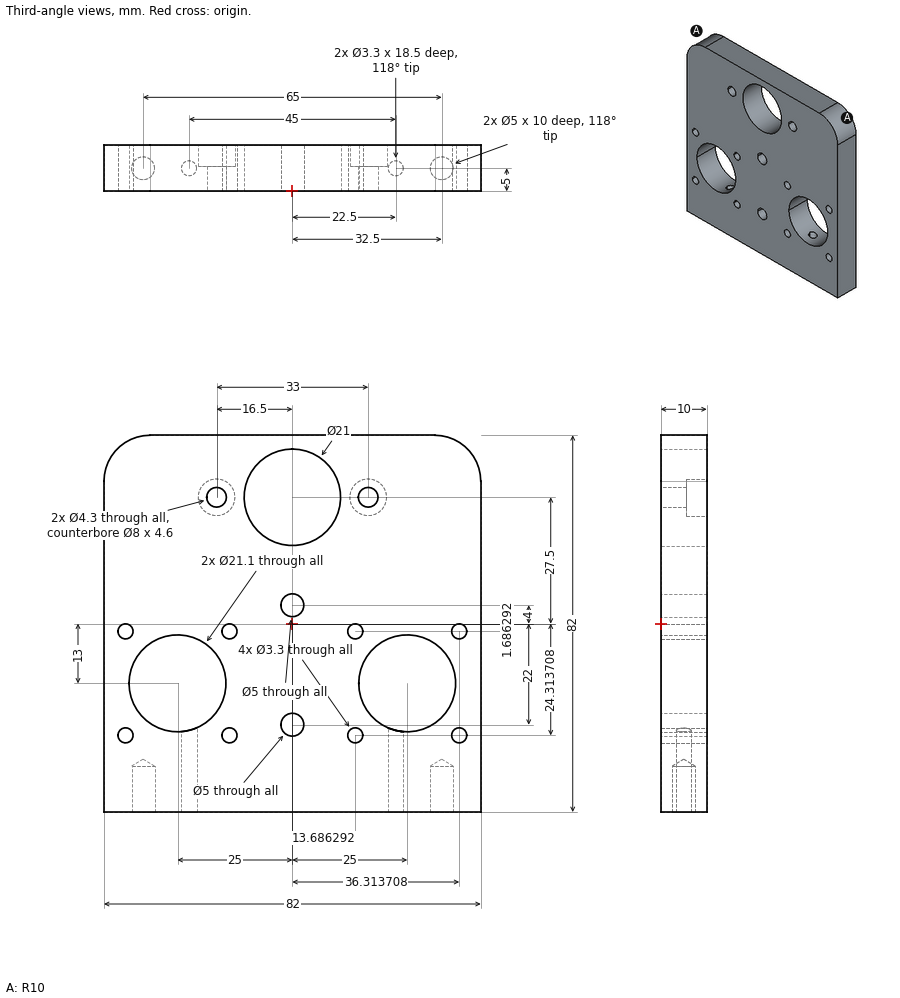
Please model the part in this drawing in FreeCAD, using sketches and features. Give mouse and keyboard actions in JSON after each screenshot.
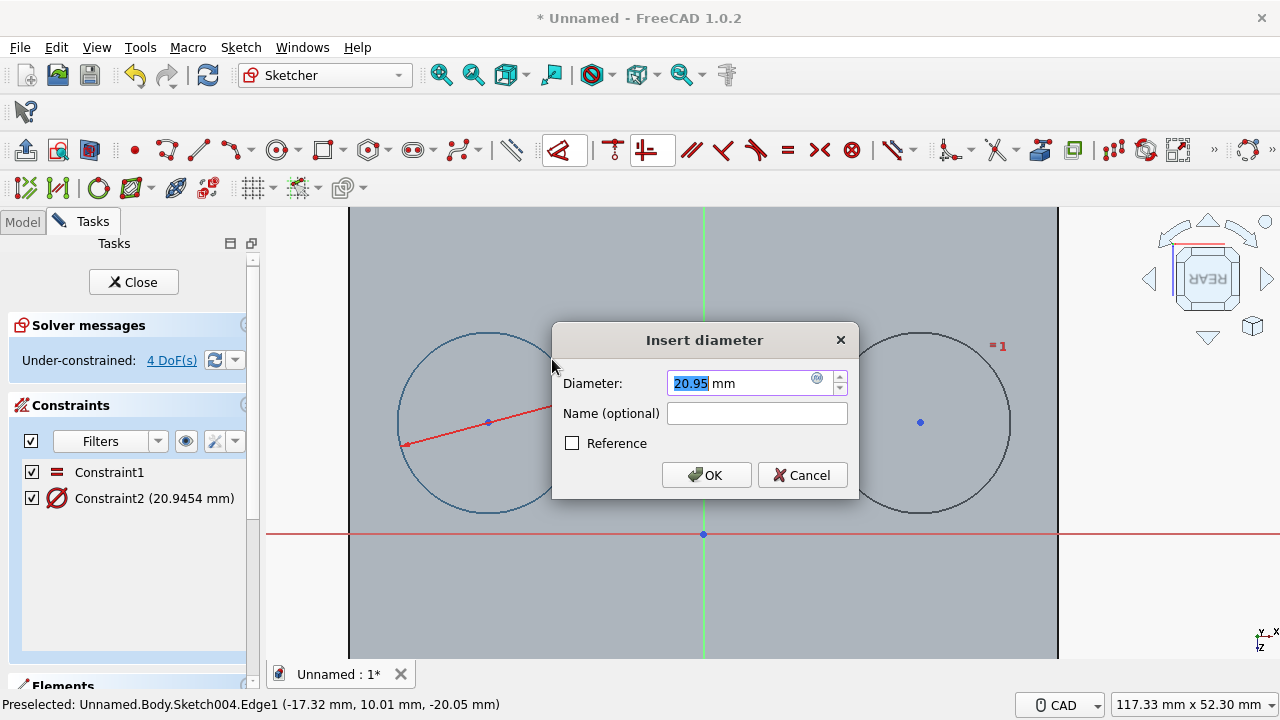
{"action": "type", "text": "21.1"}
{"action": "key", "text": "Return"}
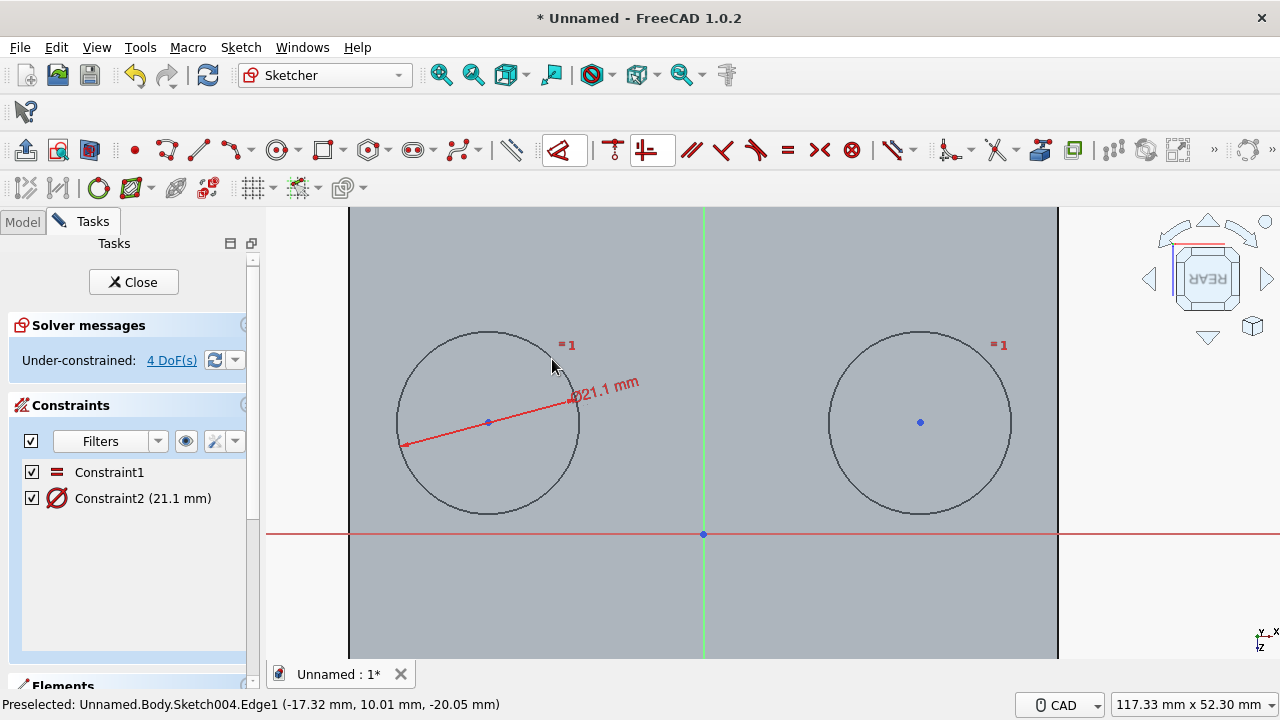
{"action": "left_click", "coordinate": [488, 423]}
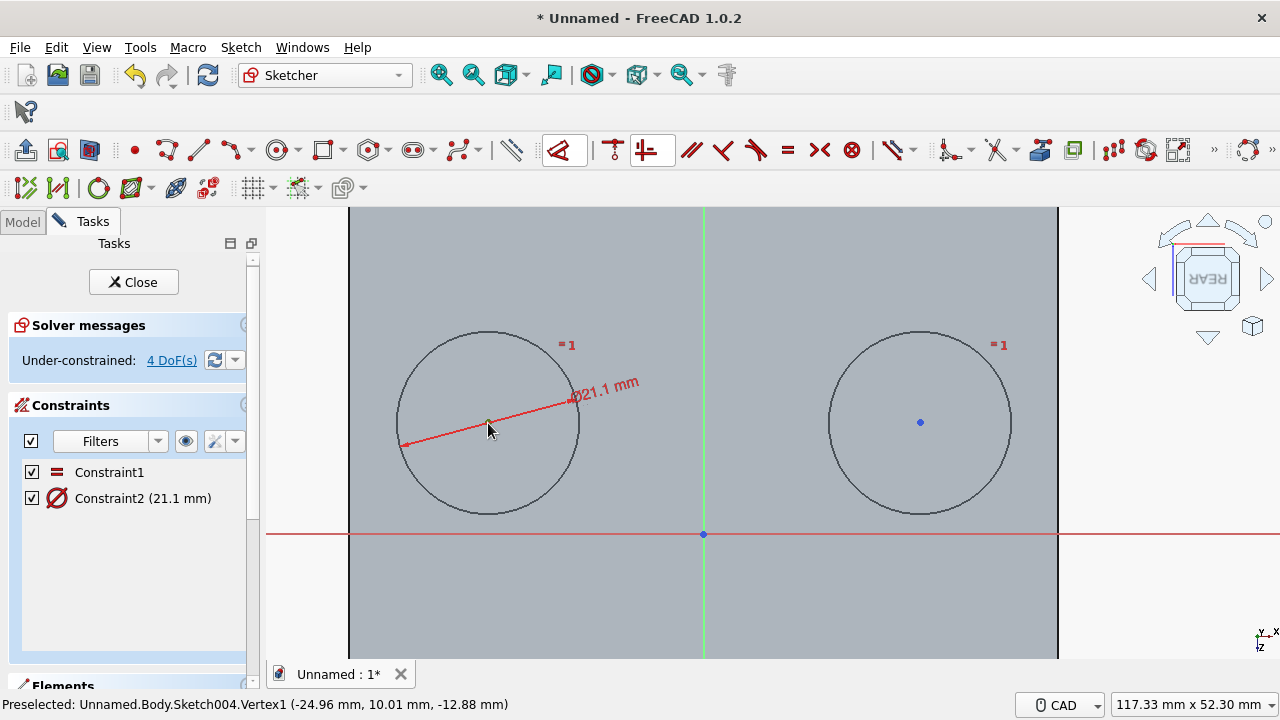
{"action": "key", "text": "l"}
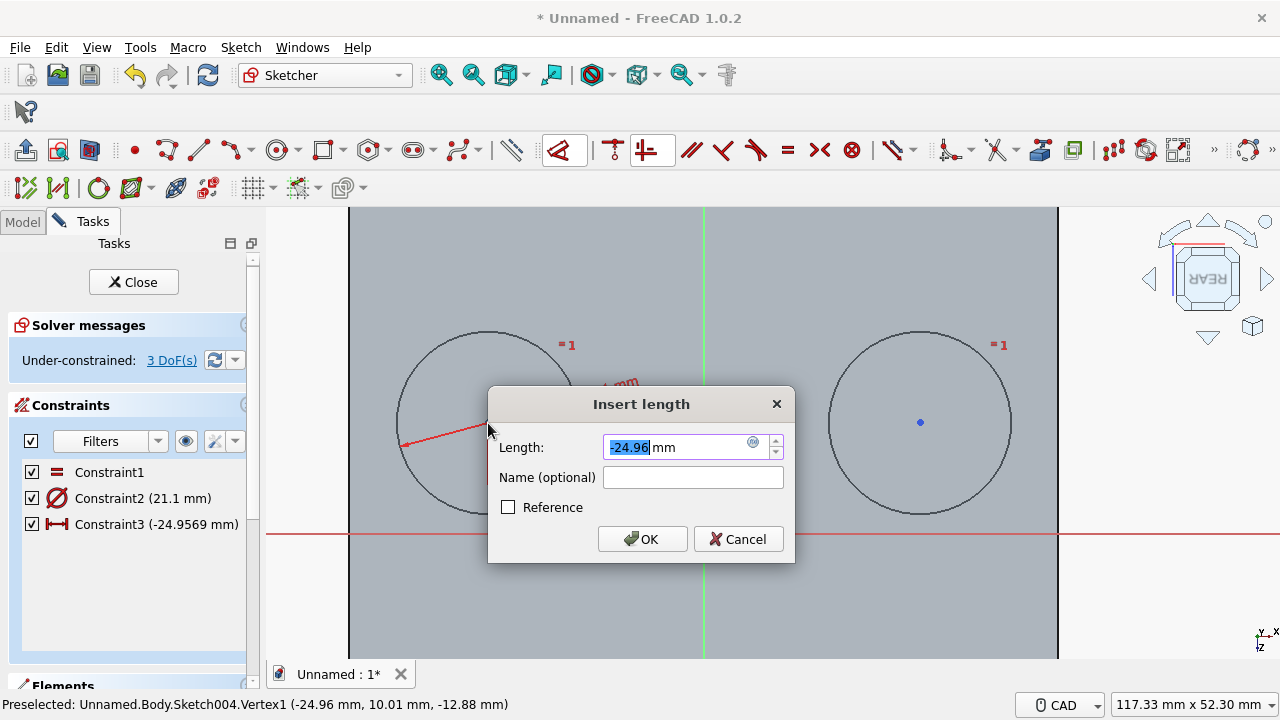
{"action": "type", "text": "-25"}
{"action": "key", "text": "Return"}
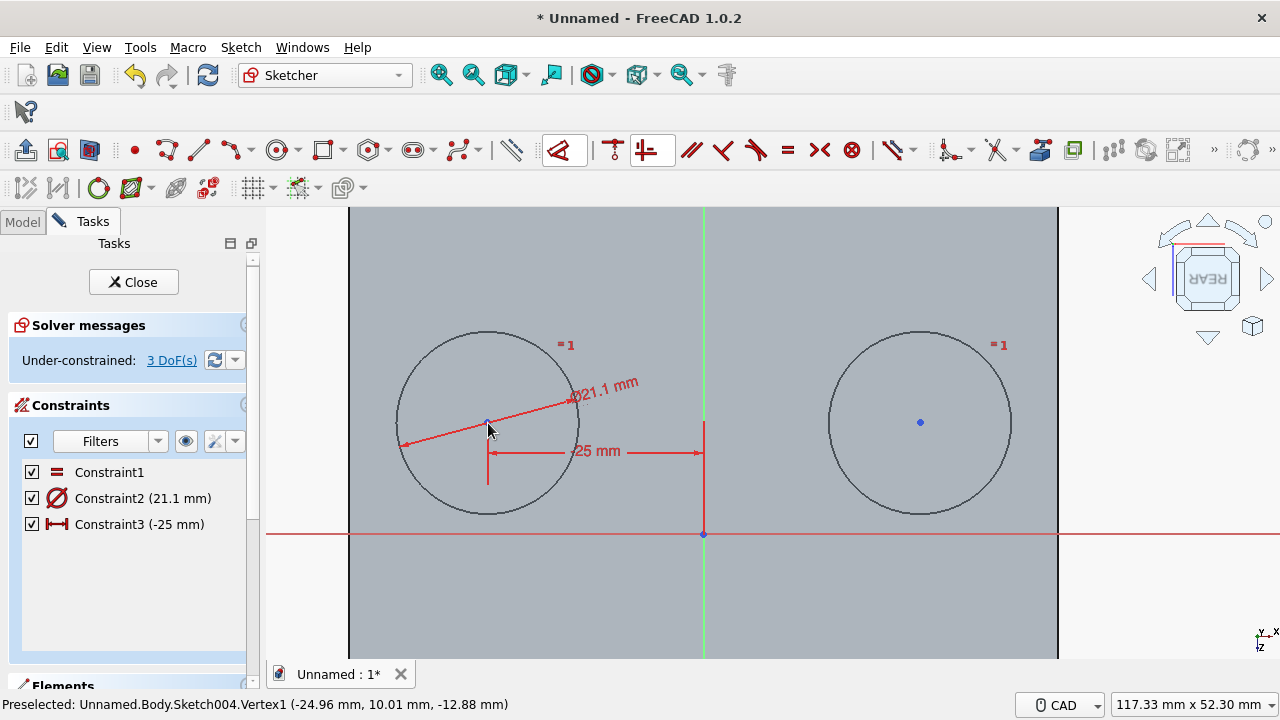
{"action": "left_click", "coordinate": [488, 423]}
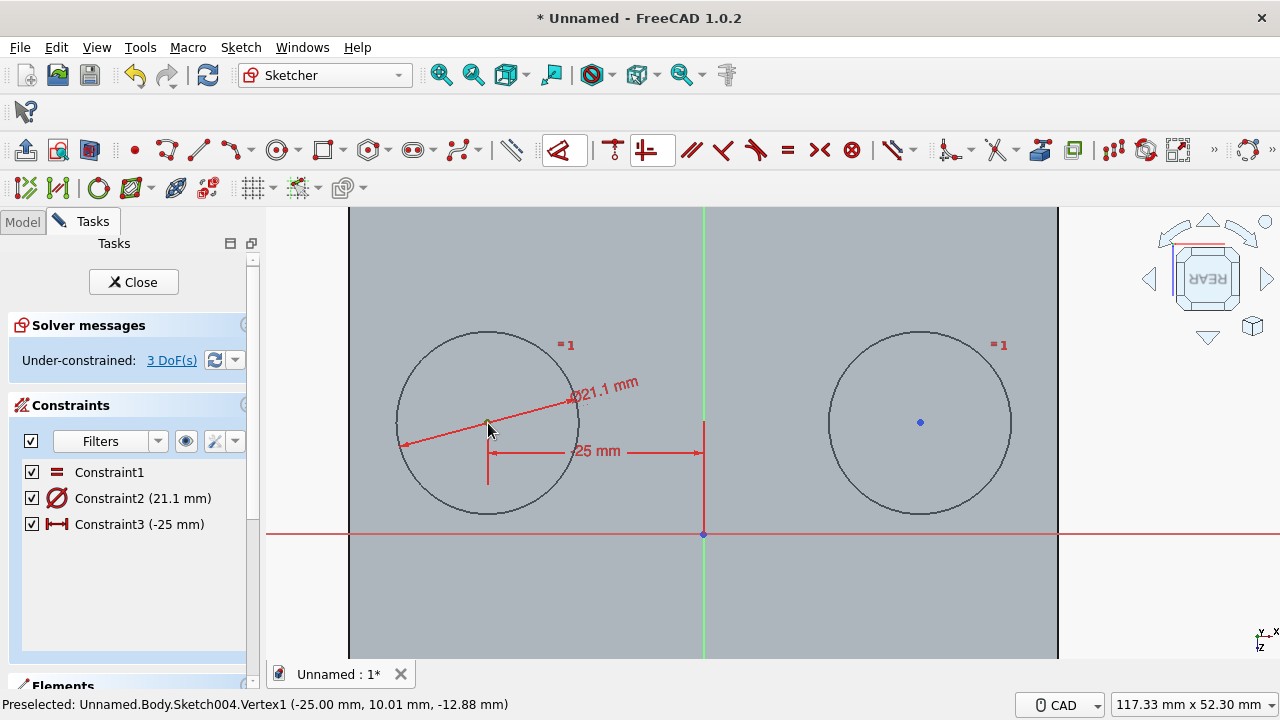
{"action": "key", "text": "i"}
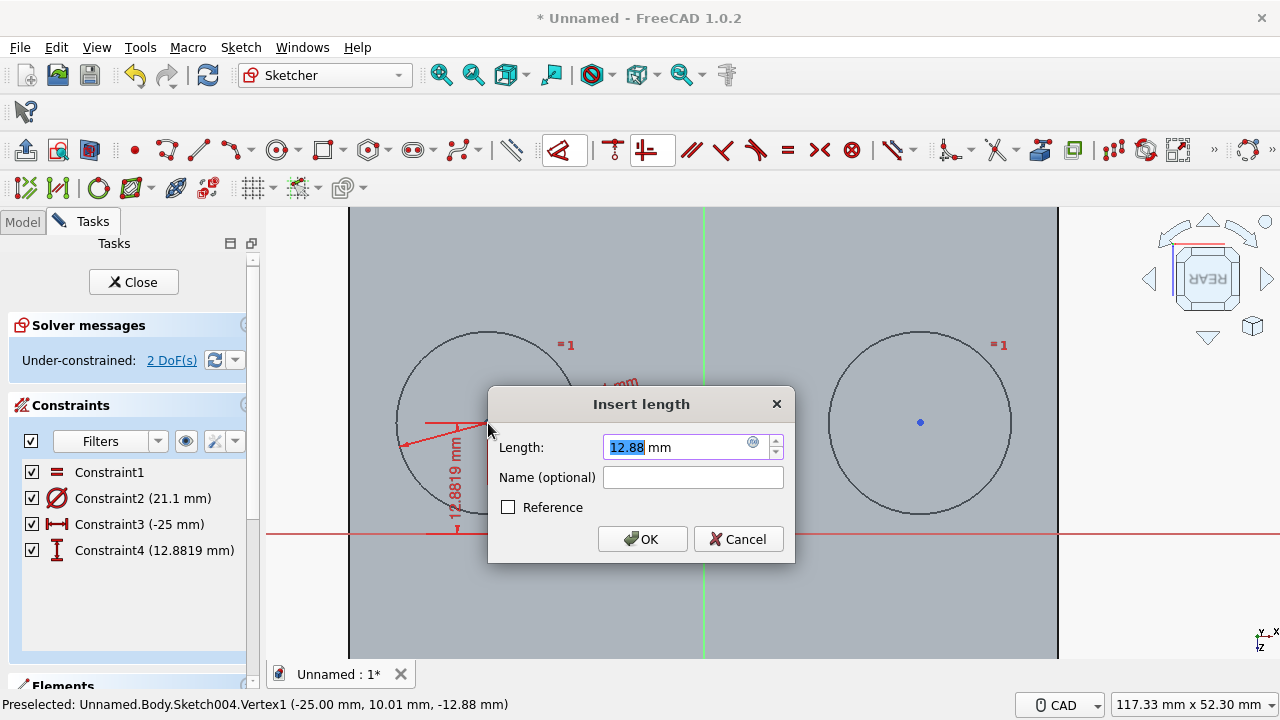
{"action": "type", "text": "13"}
{"action": "key", "text": "Return"}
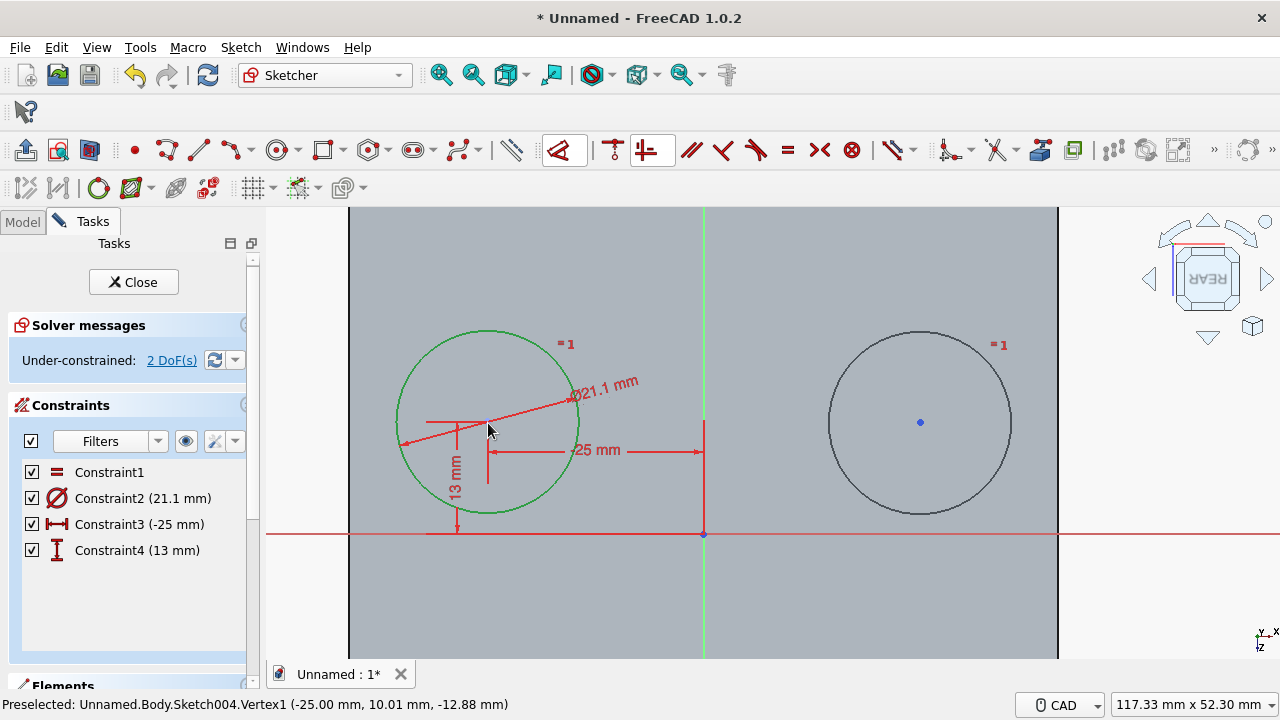
{"action": "left_click", "coordinate": [920, 423]}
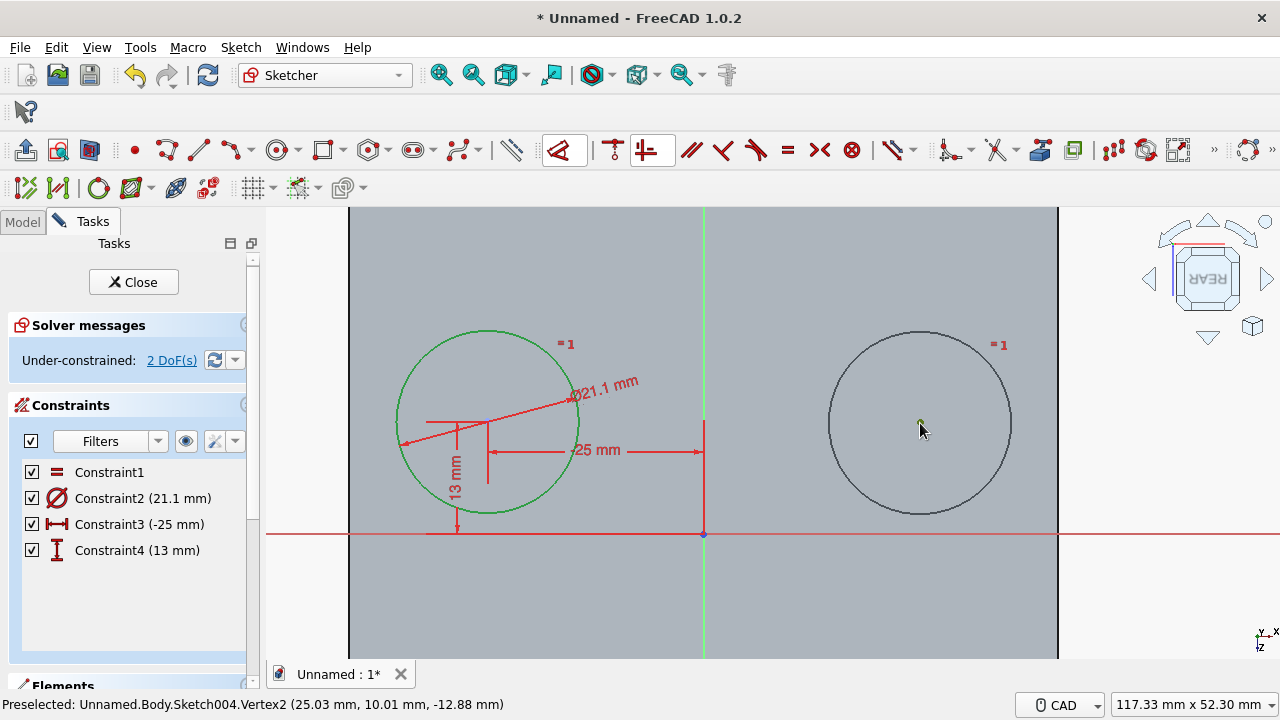
{"action": "key", "text": "l"}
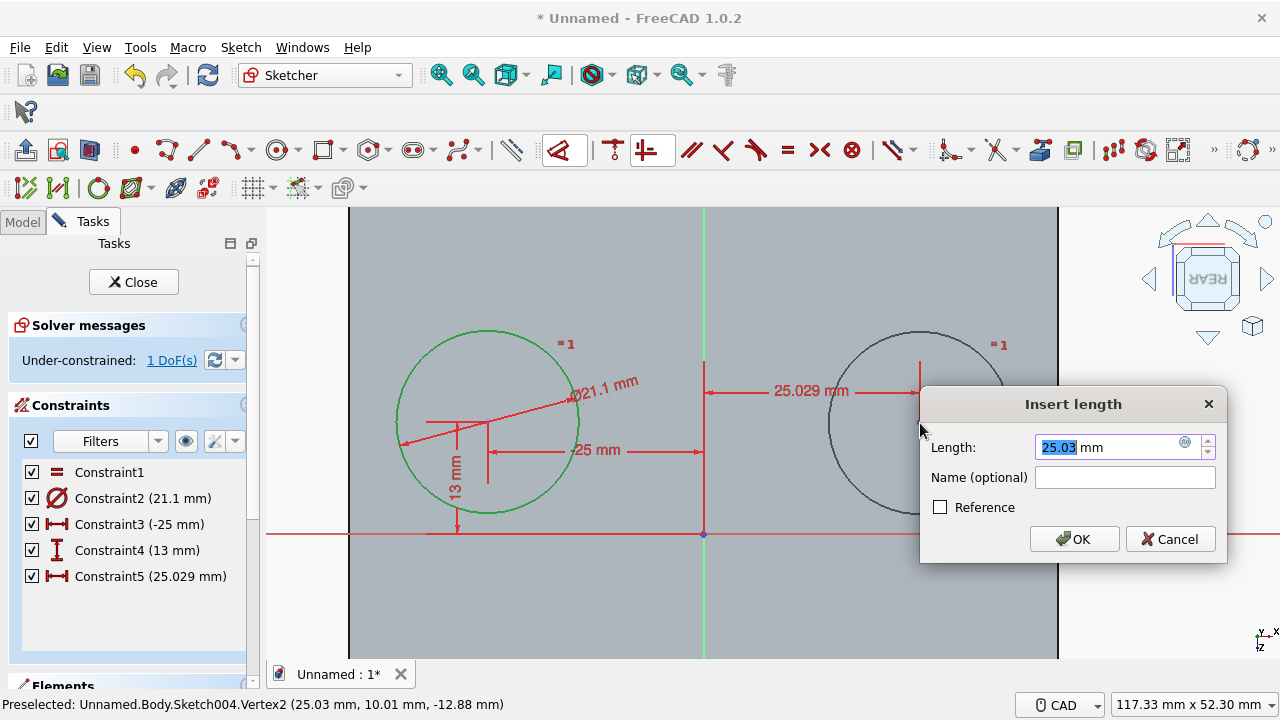
{"action": "type", "text": "25"}
{"action": "key", "text": "Return"}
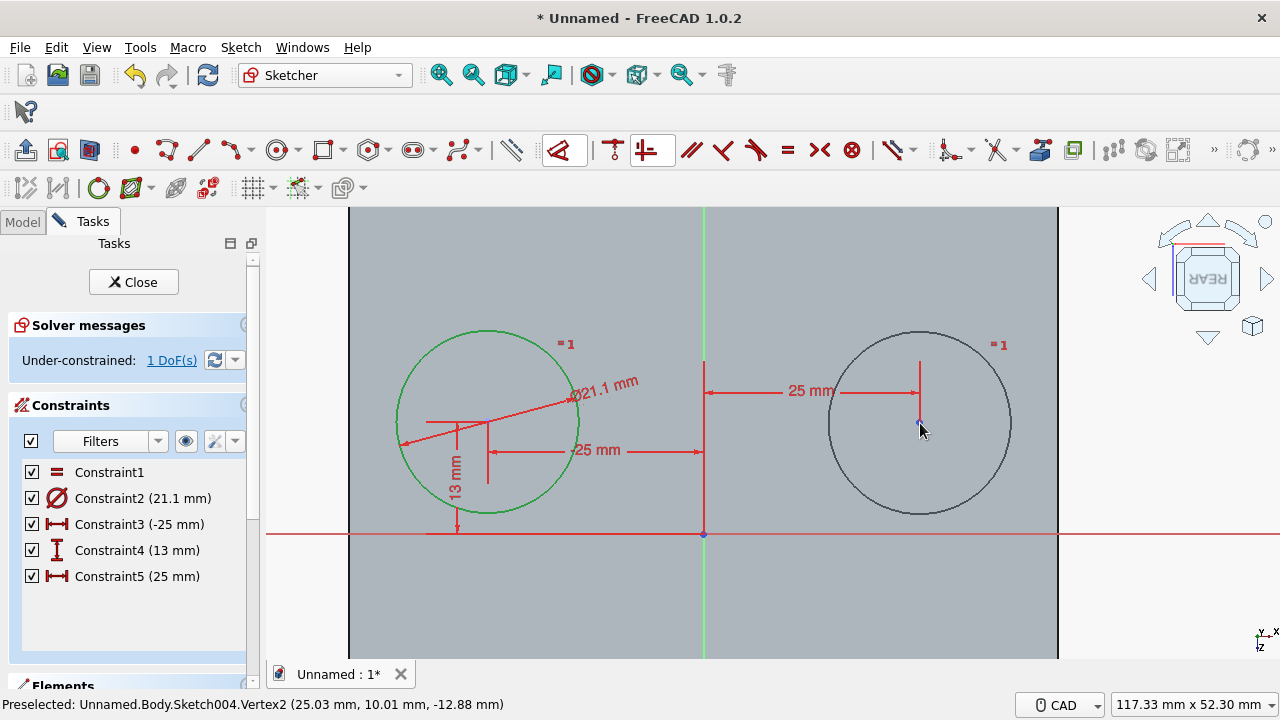
{"action": "left_click", "coordinate": [920, 423]}